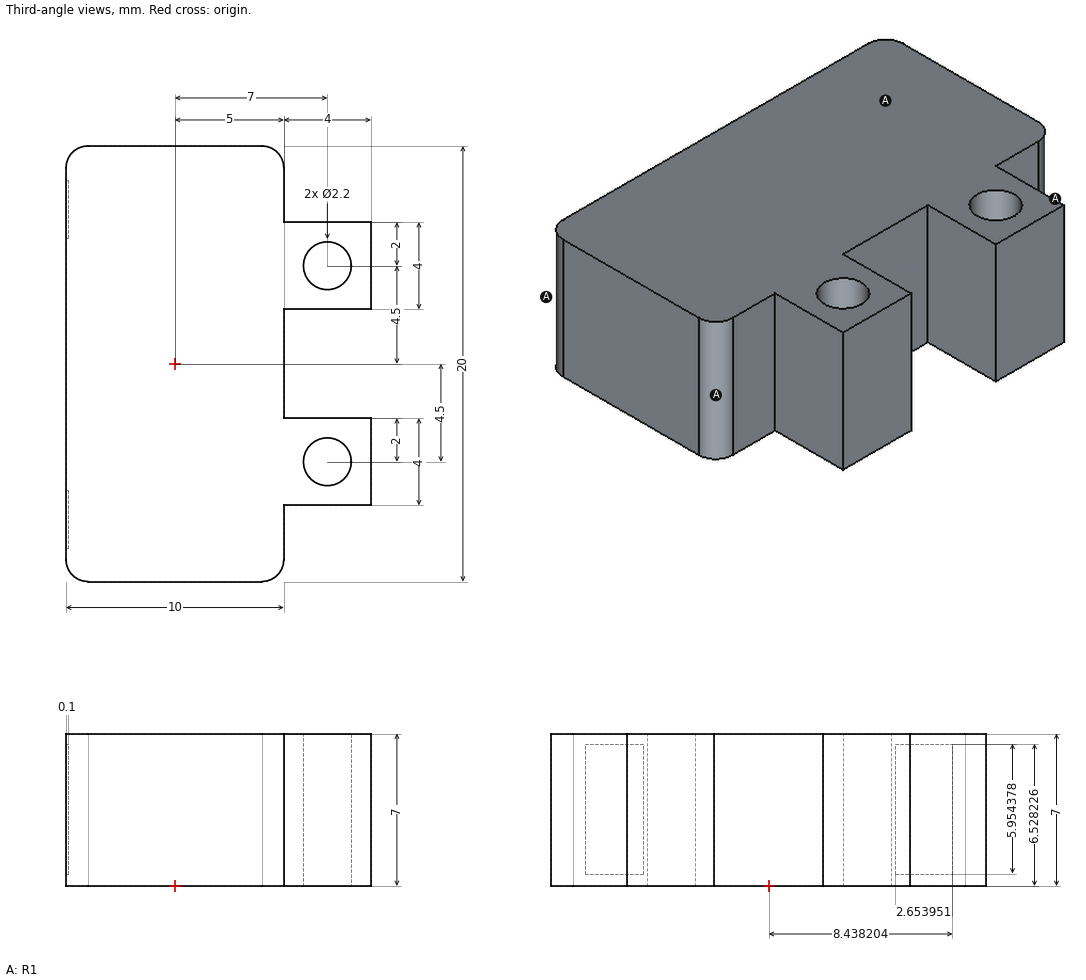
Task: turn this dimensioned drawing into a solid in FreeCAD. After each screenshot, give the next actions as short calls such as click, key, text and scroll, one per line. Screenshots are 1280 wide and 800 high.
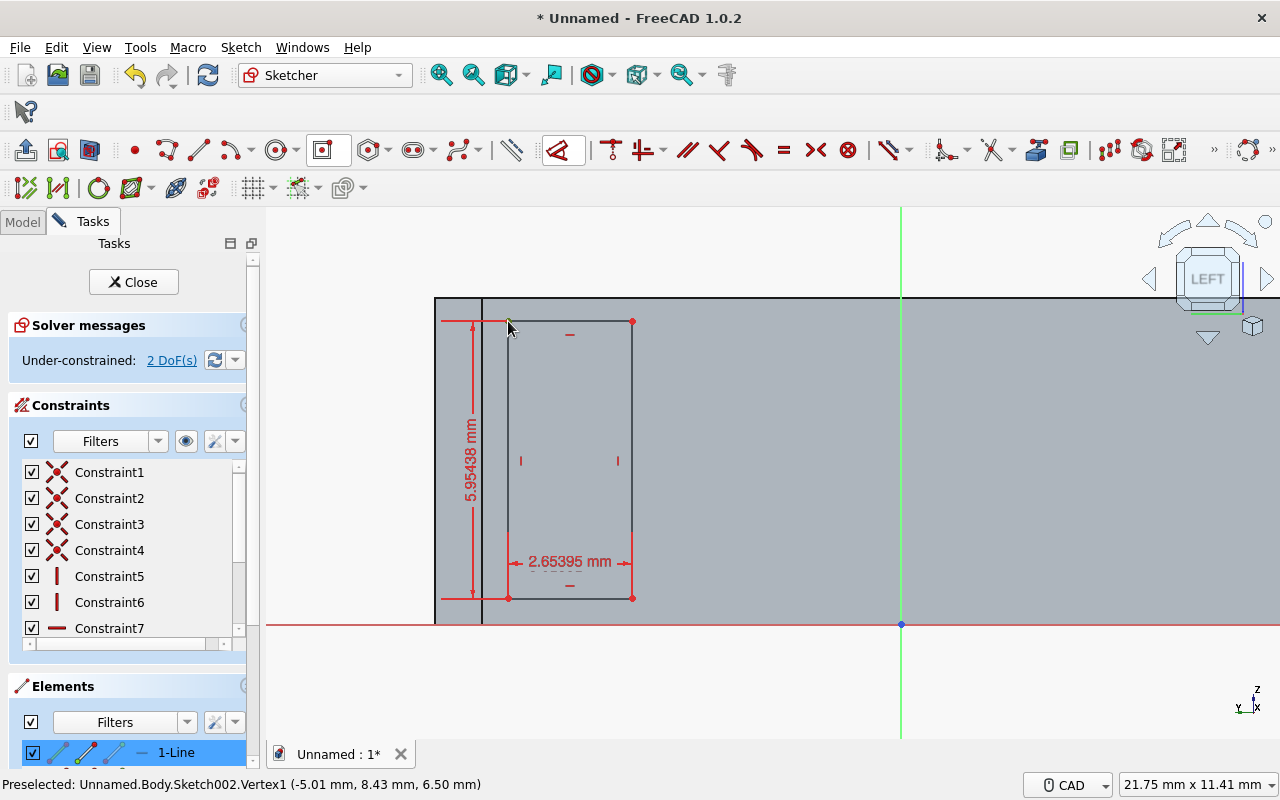
key(l)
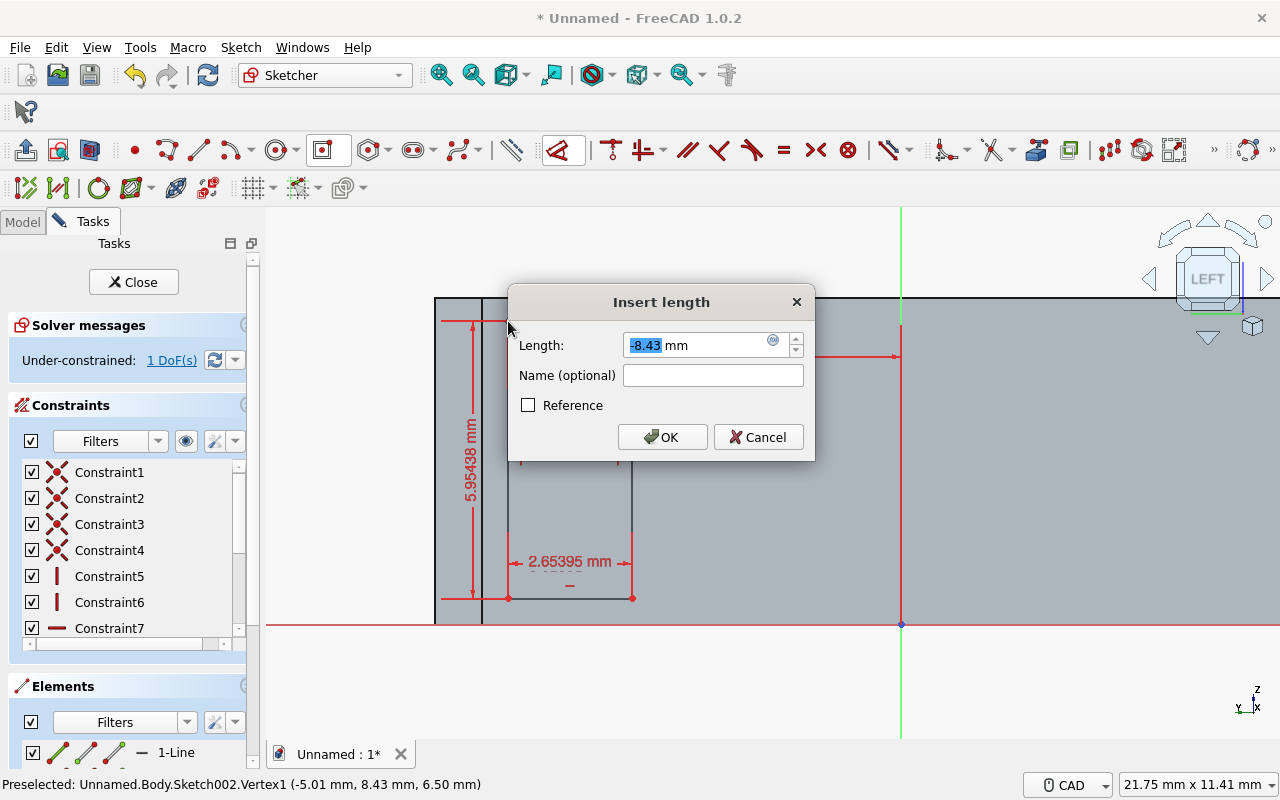
text(-8.438204)
key(Return)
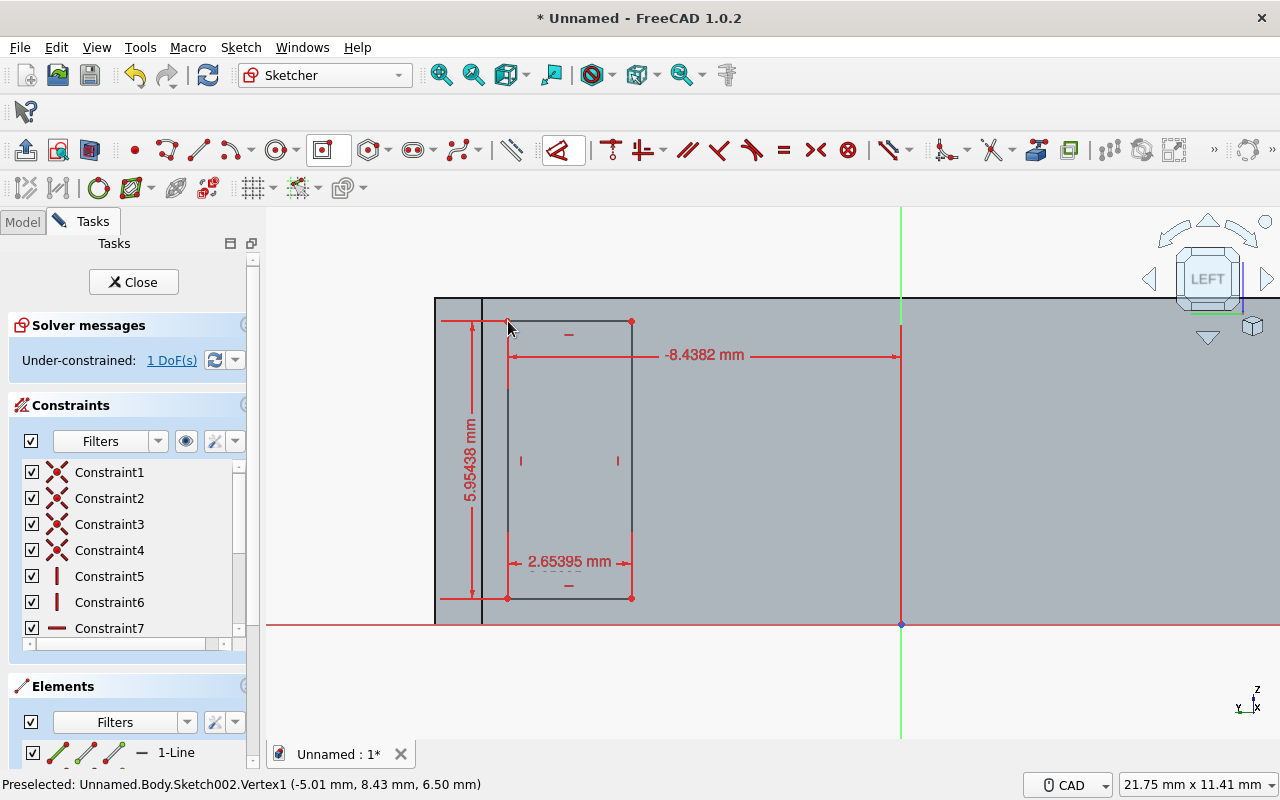
click(508, 321)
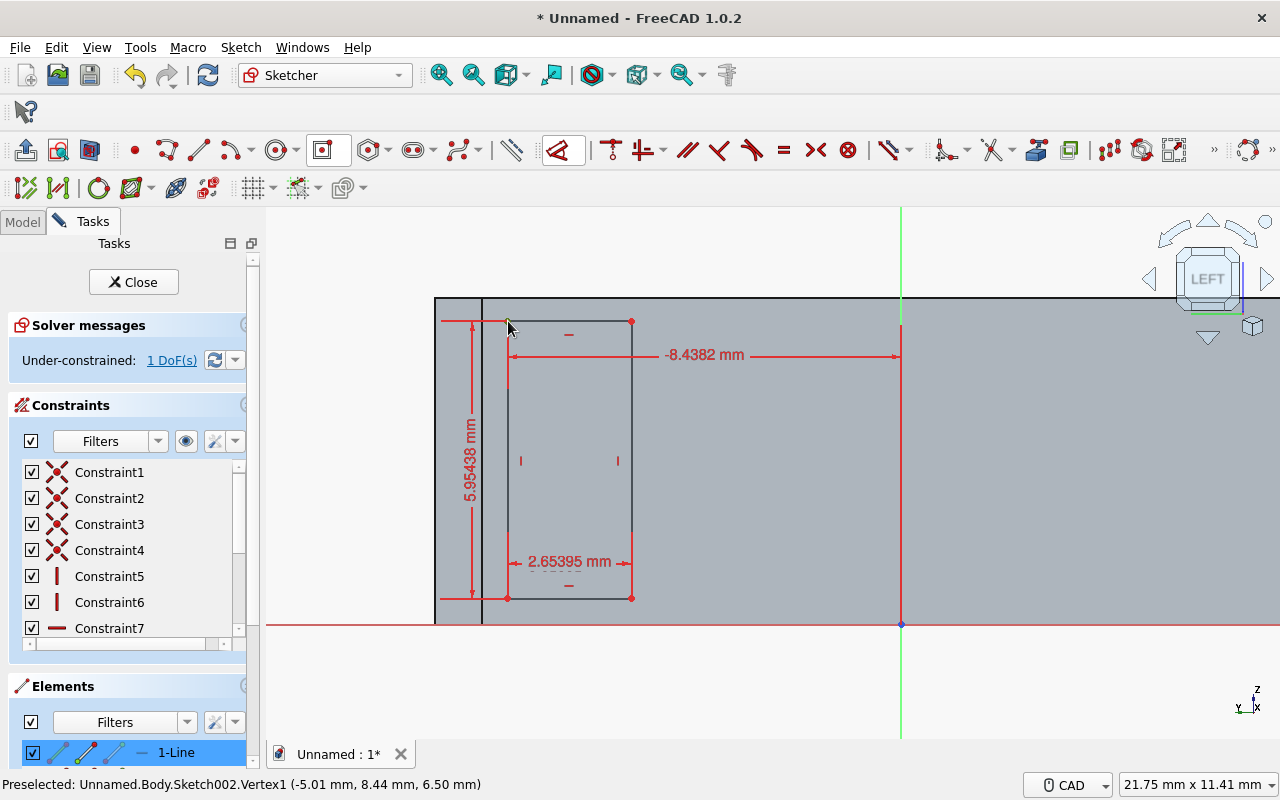
key(i)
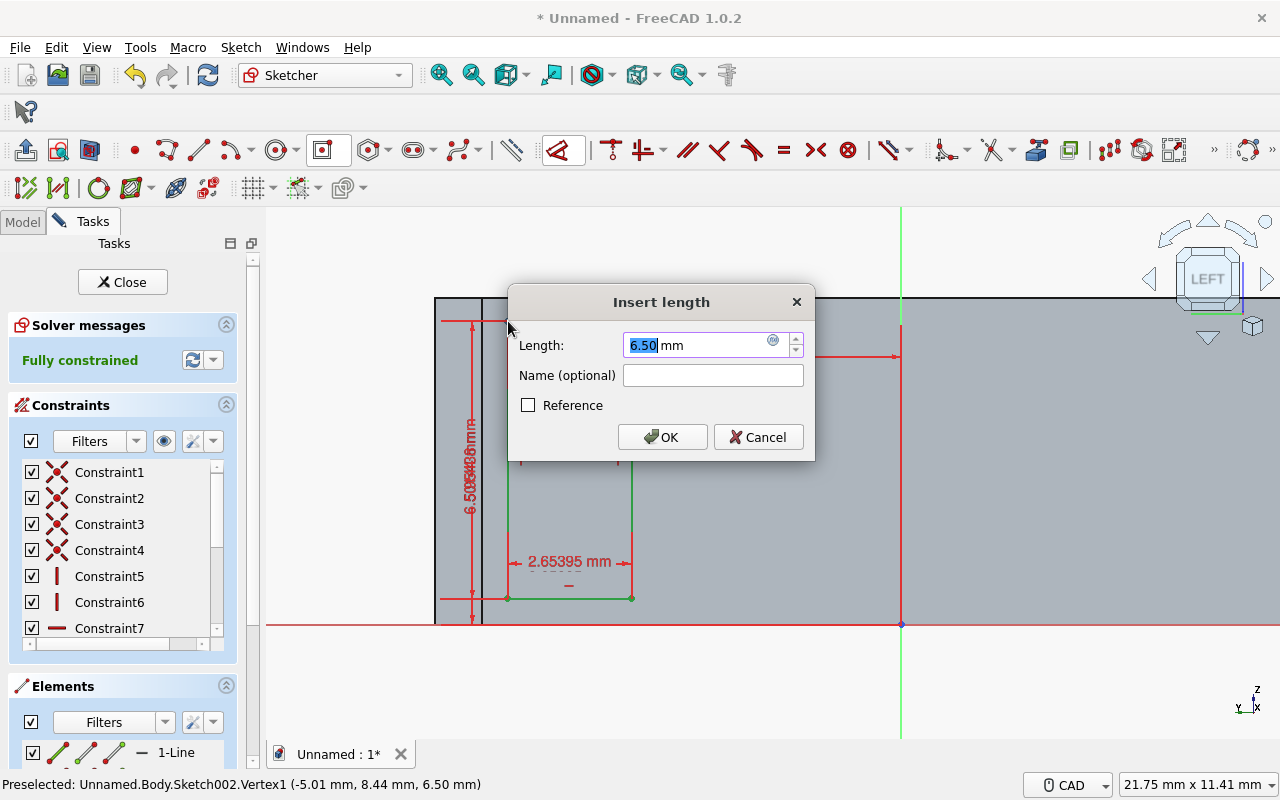
text(6.528226)
key(Return)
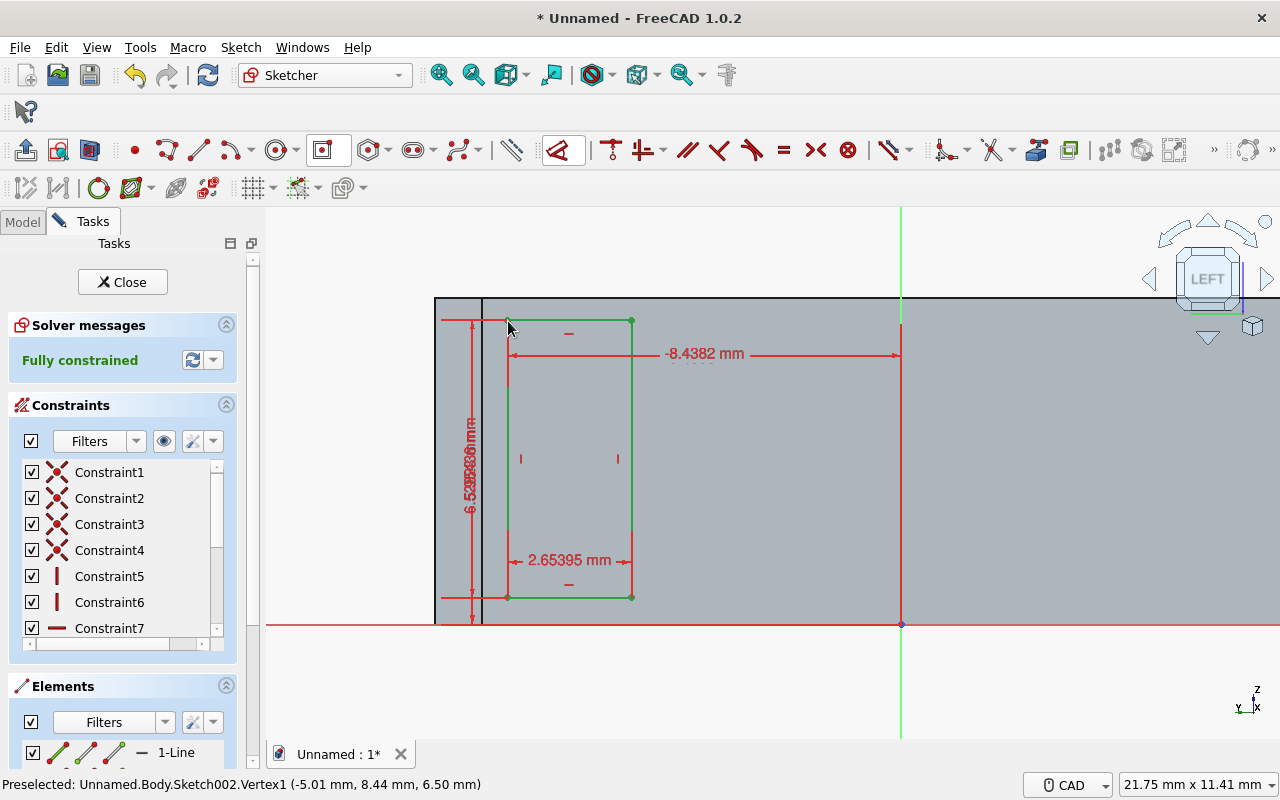
click(123, 282)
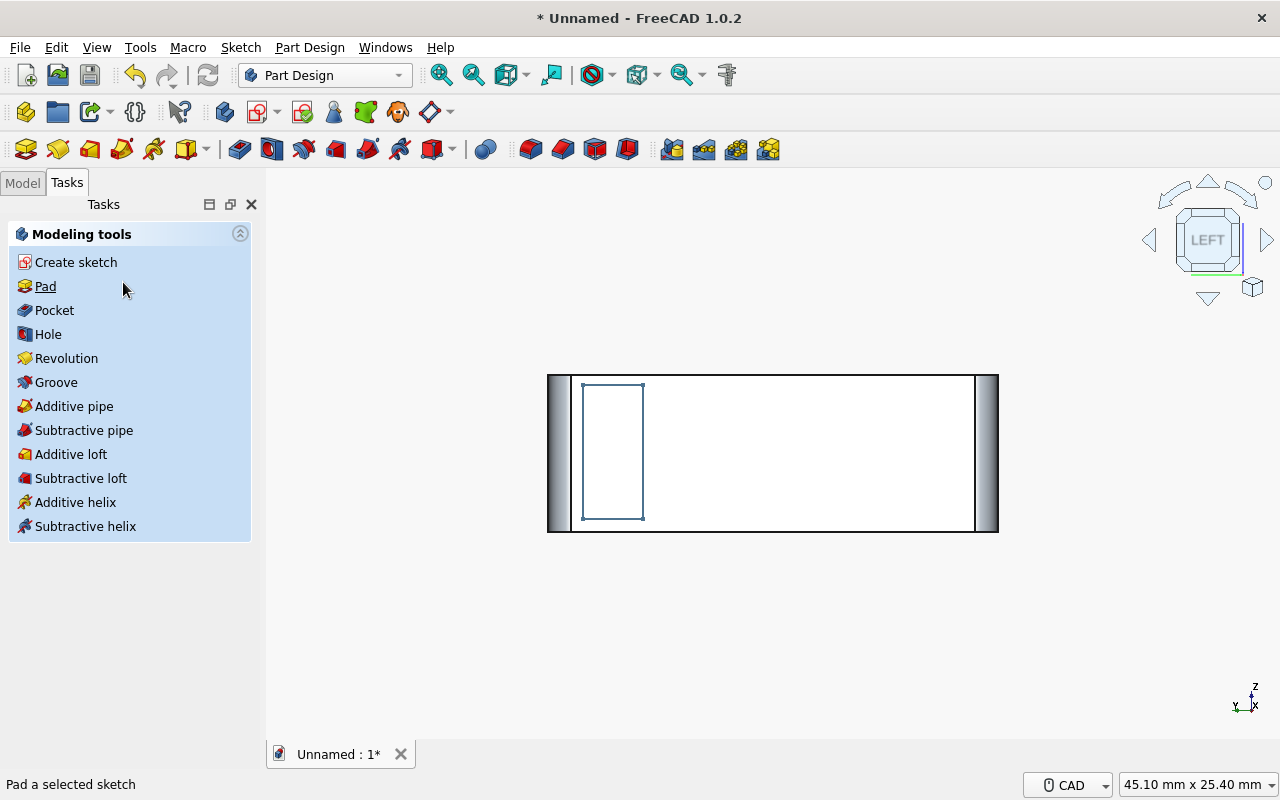
click(240, 150)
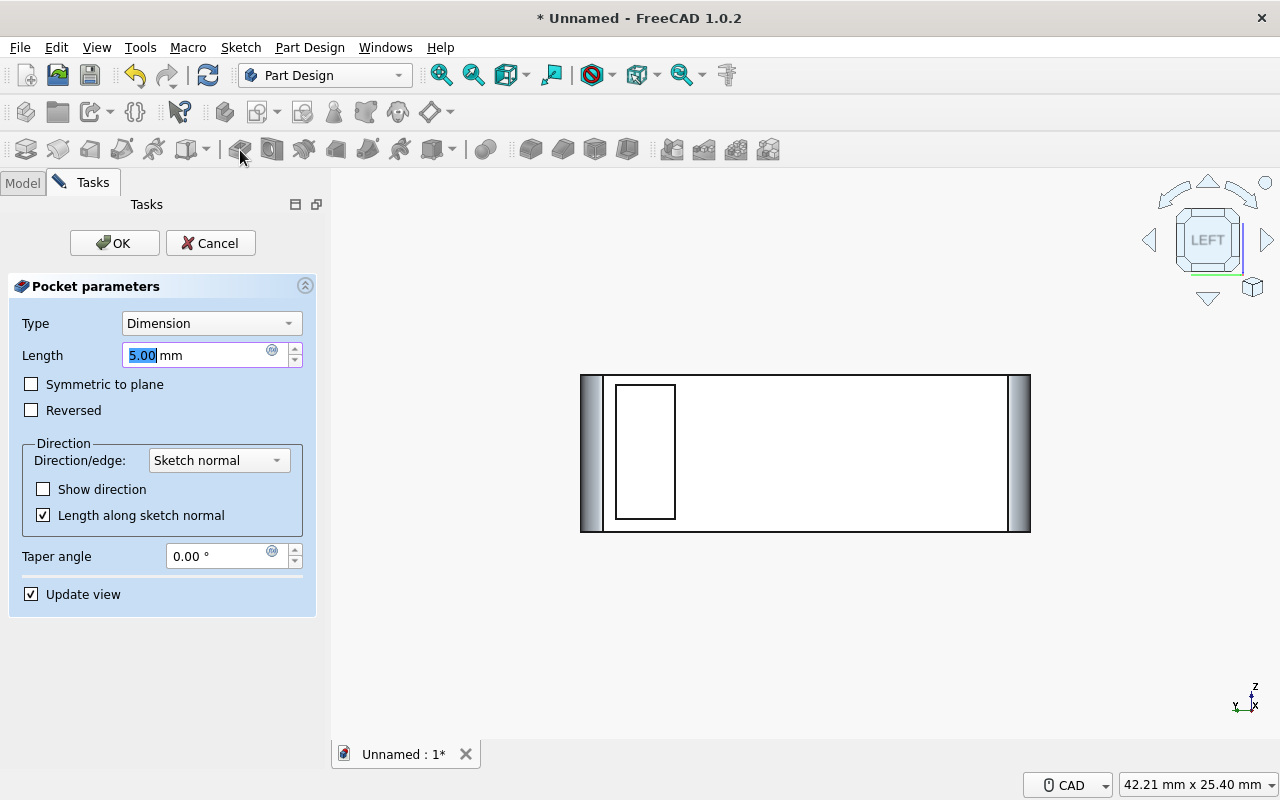
text(0.1)
key(Tab)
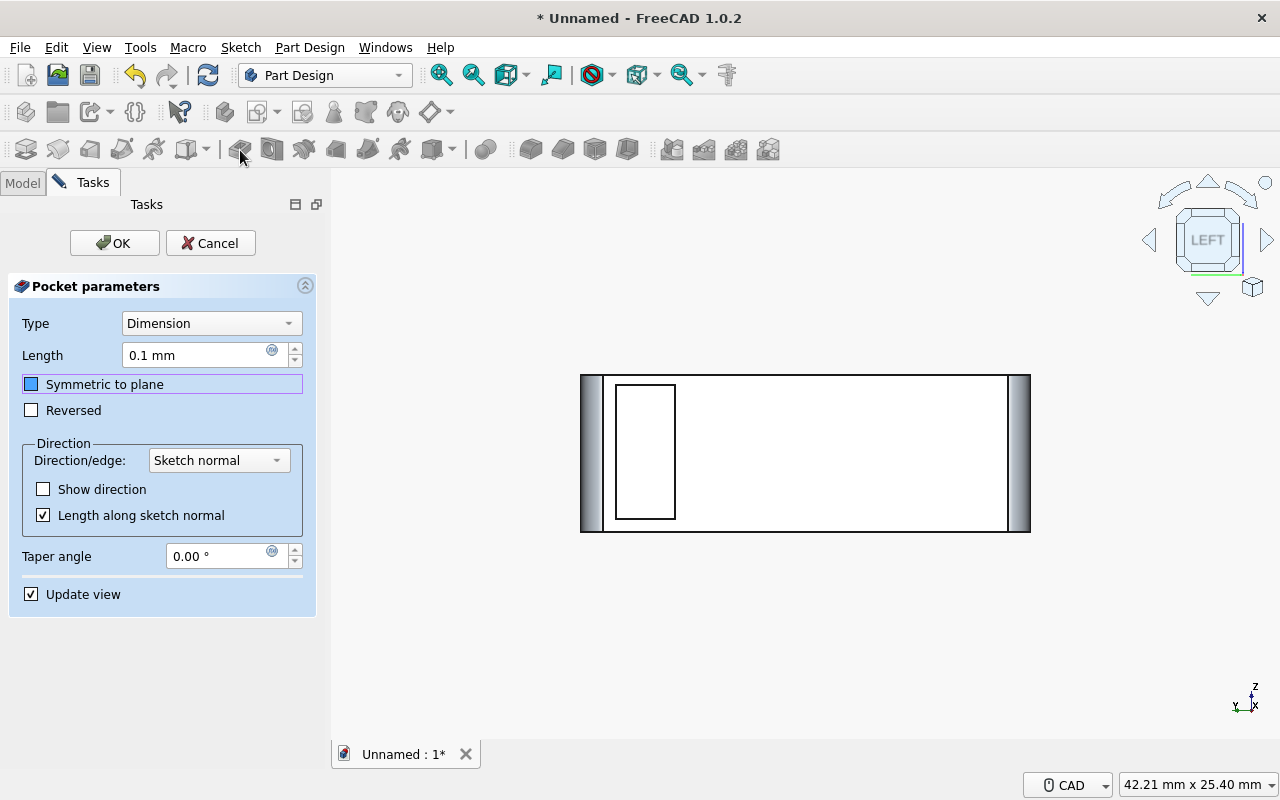
click(115, 243)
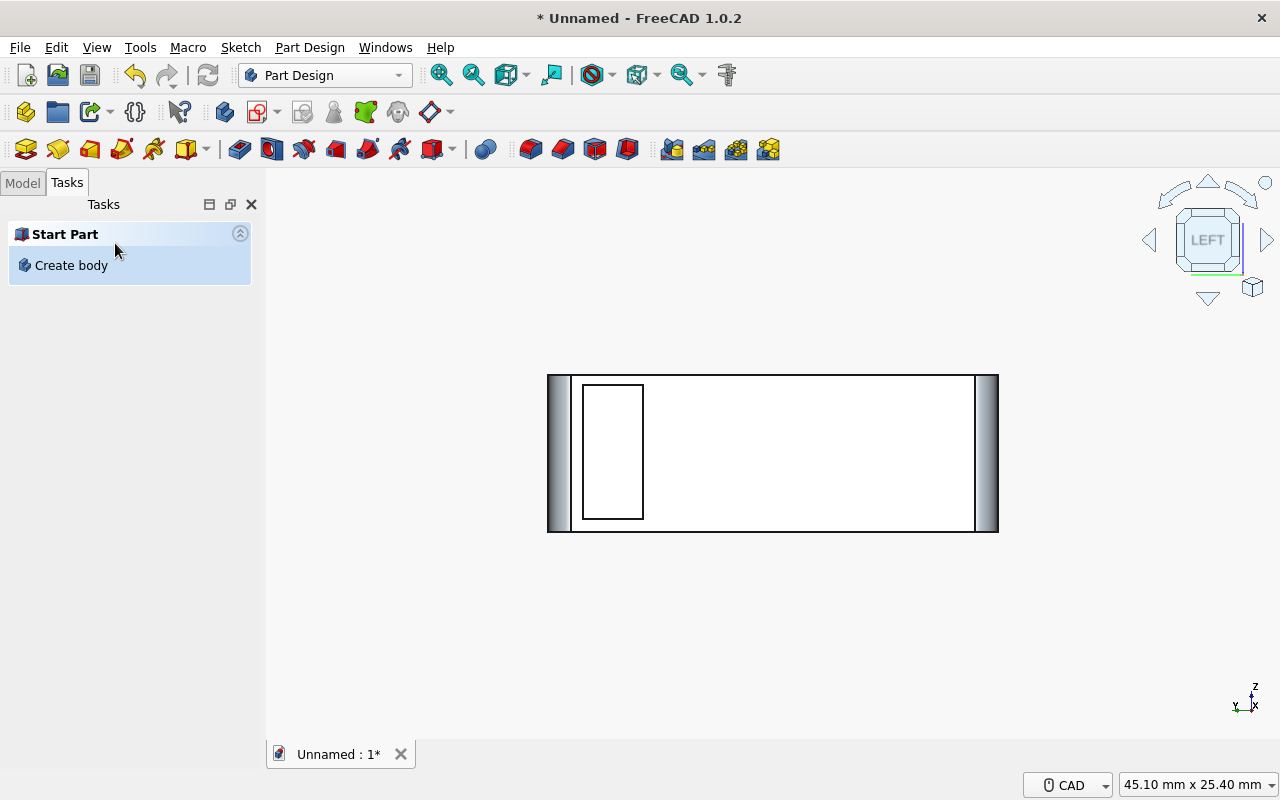
click(442, 76)